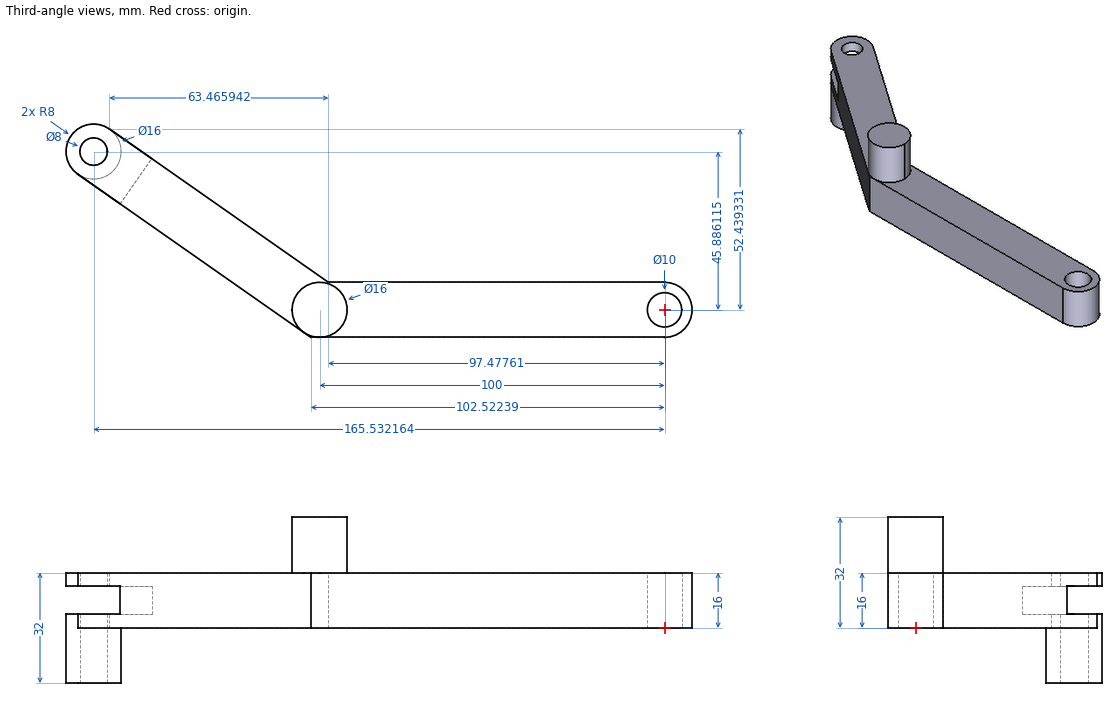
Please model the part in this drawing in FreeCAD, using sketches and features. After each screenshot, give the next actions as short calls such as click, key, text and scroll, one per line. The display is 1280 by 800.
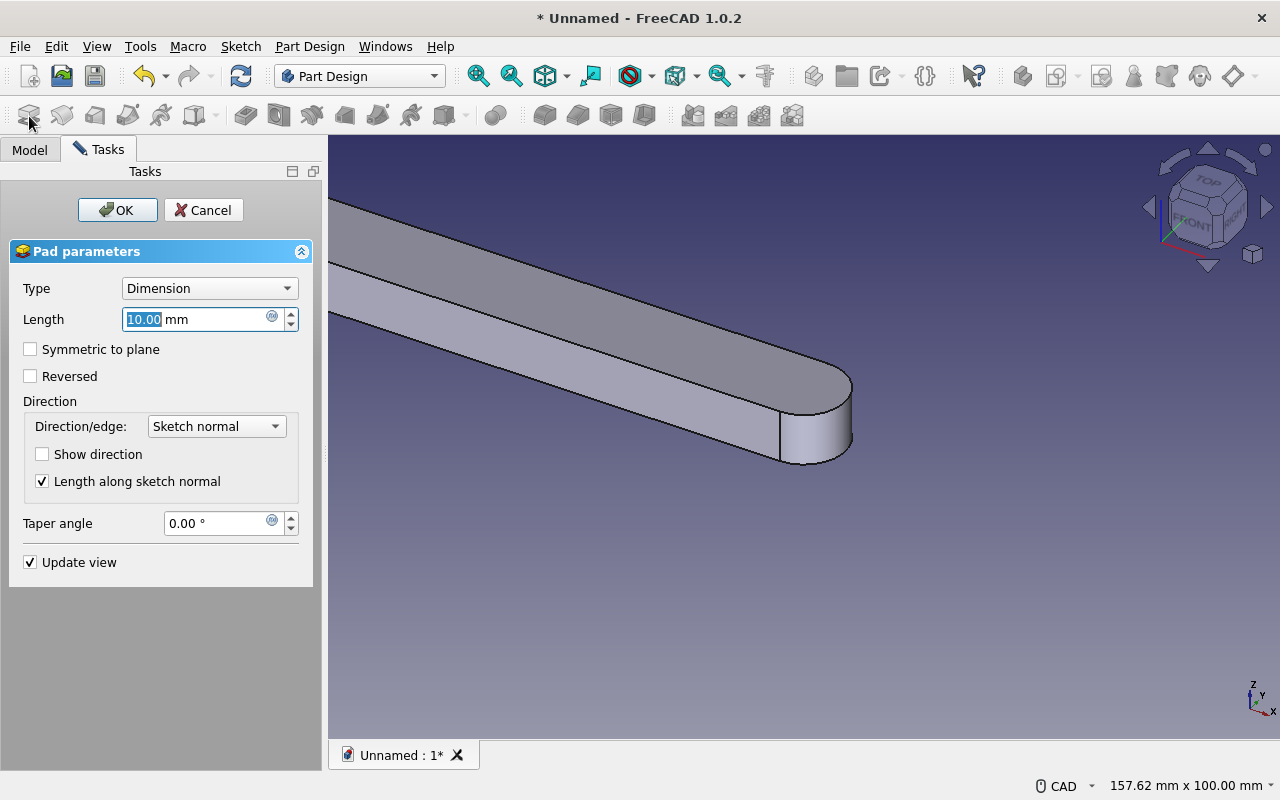
text(16)
key(Tab)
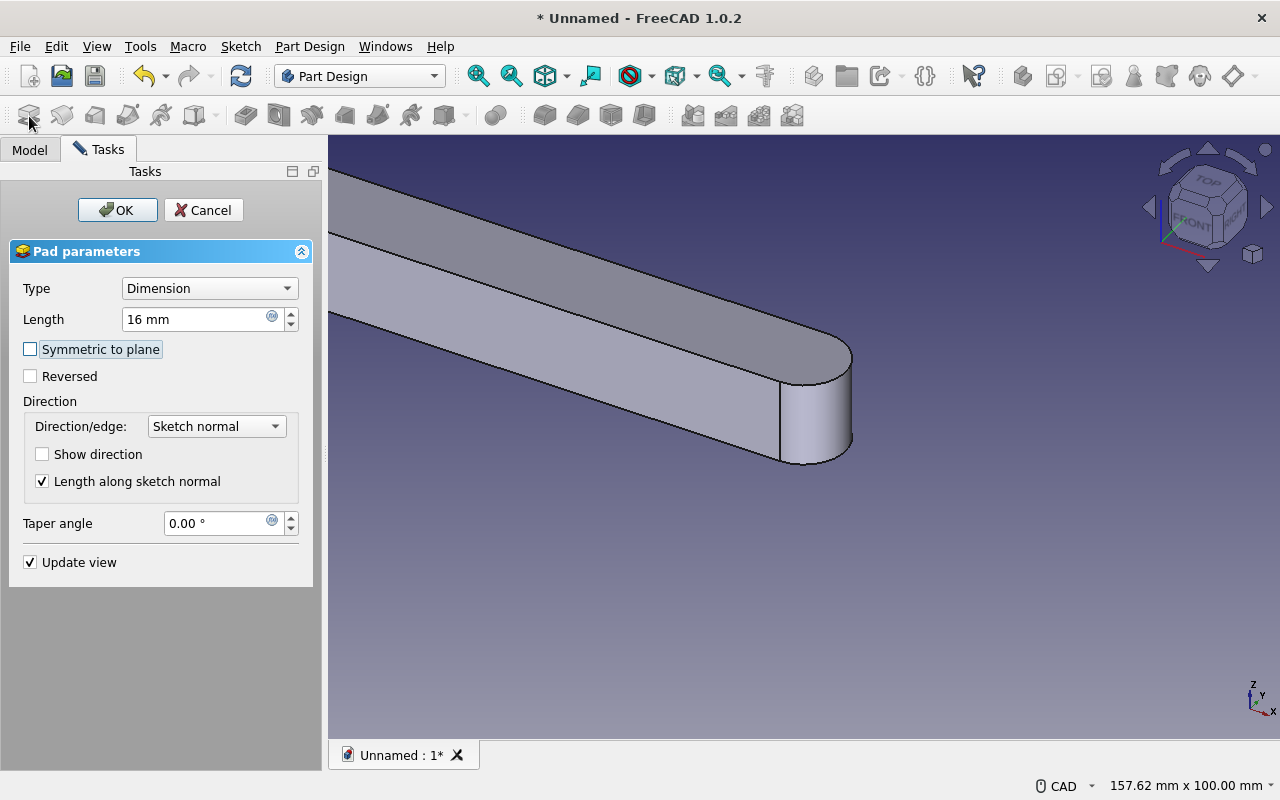
click(118, 210)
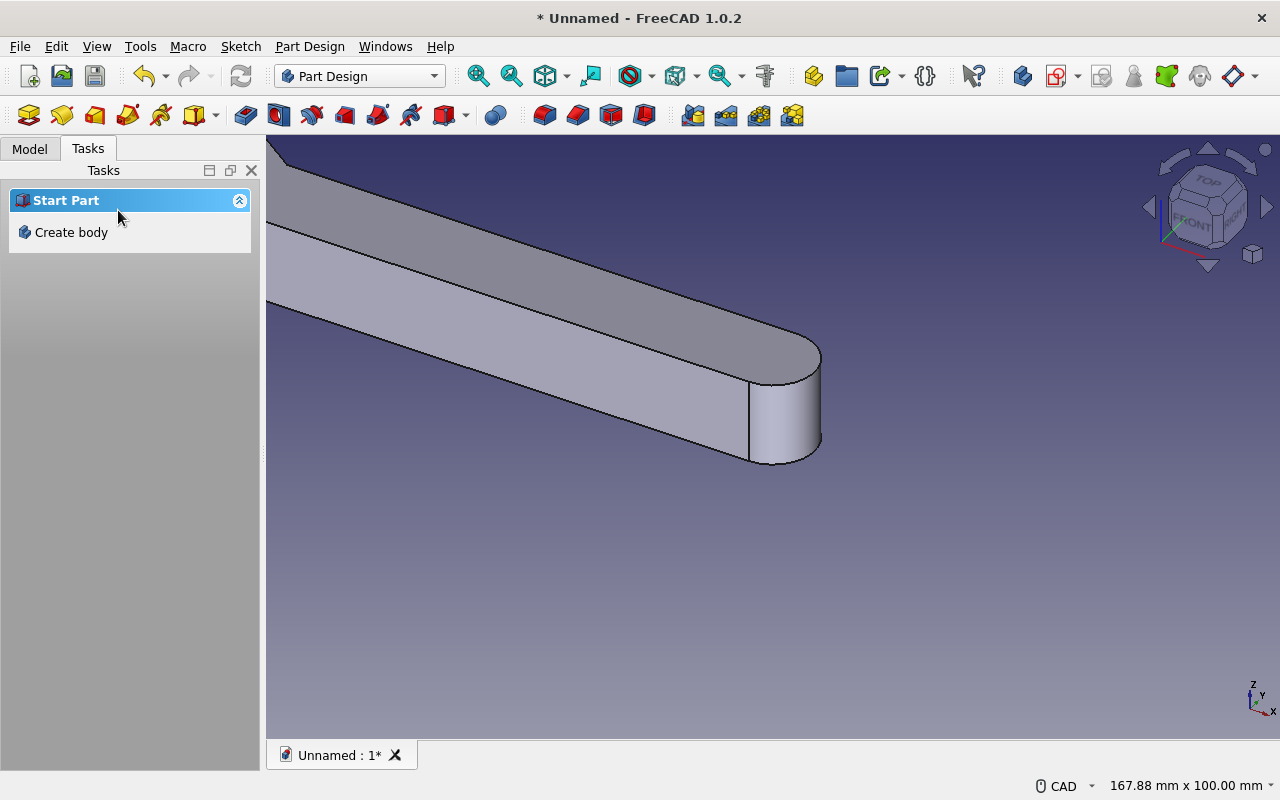
click(479, 76)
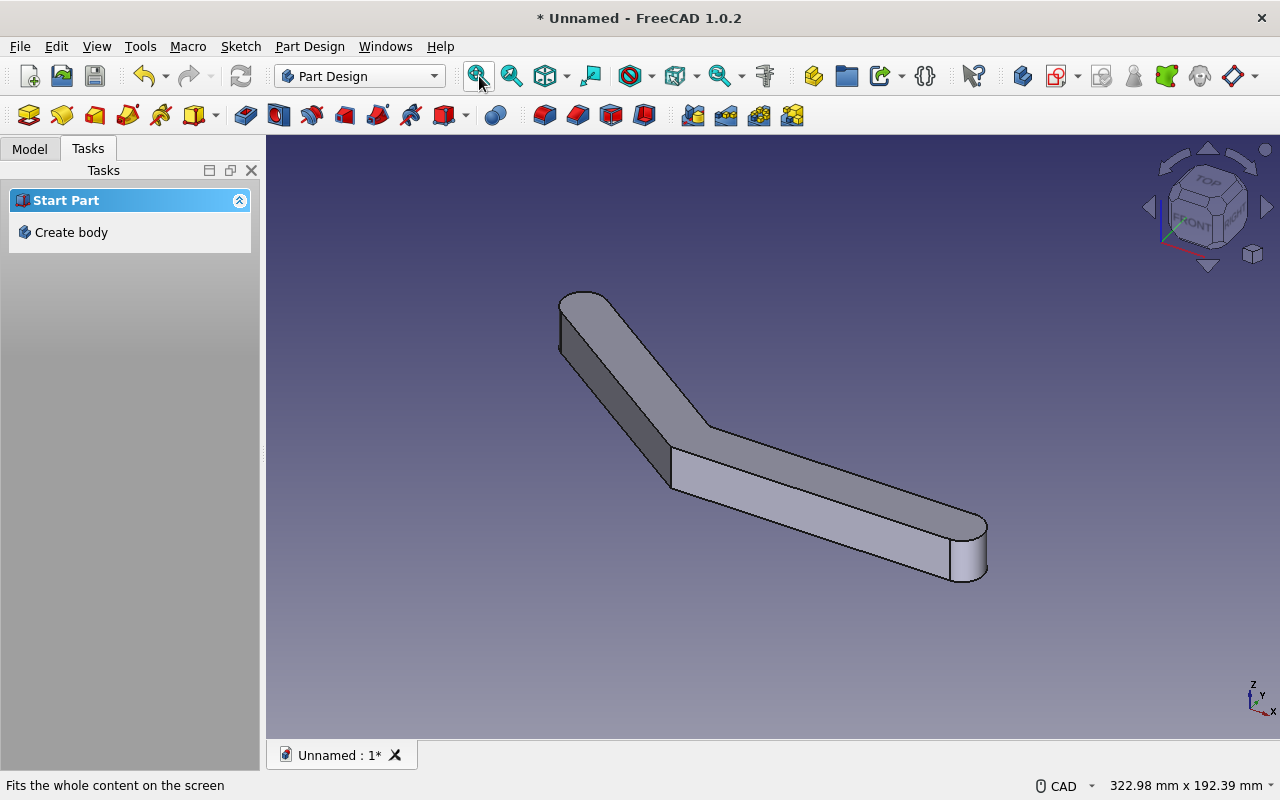
click(675, 420)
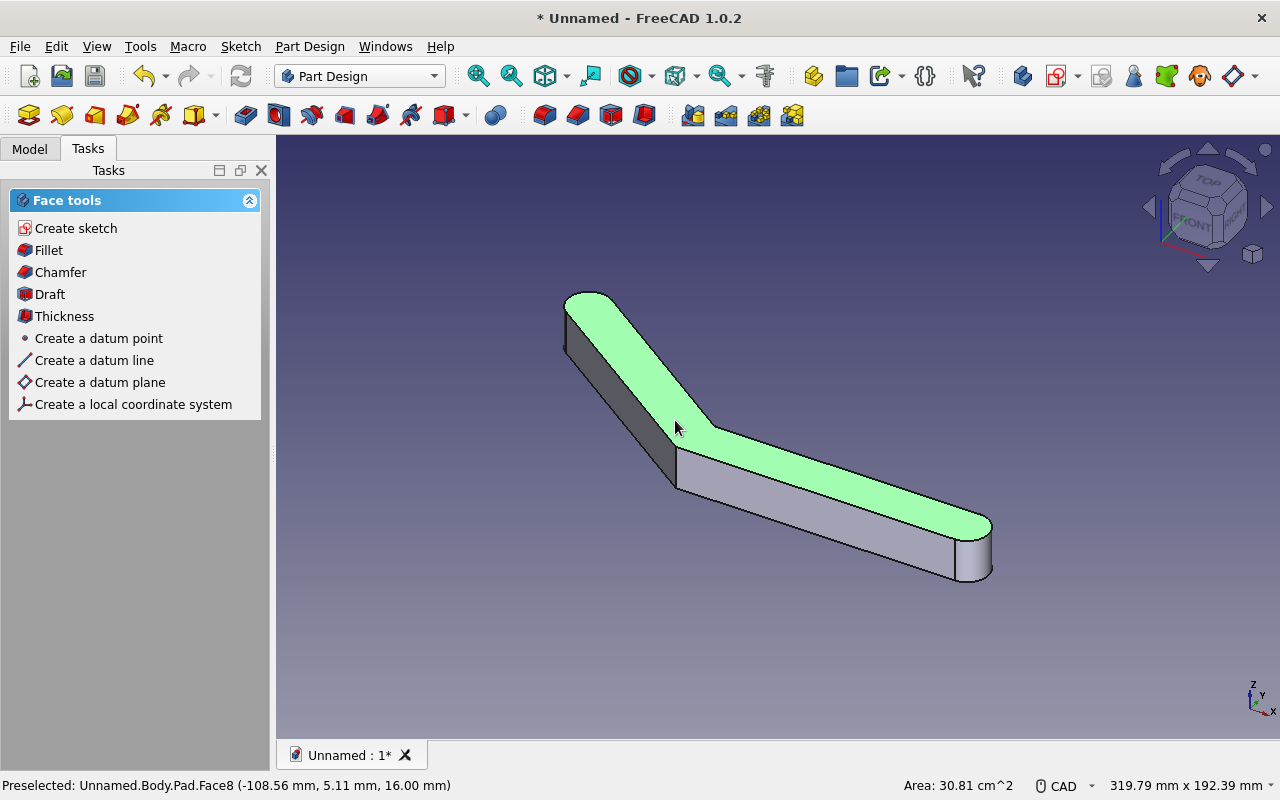
click(1056, 76)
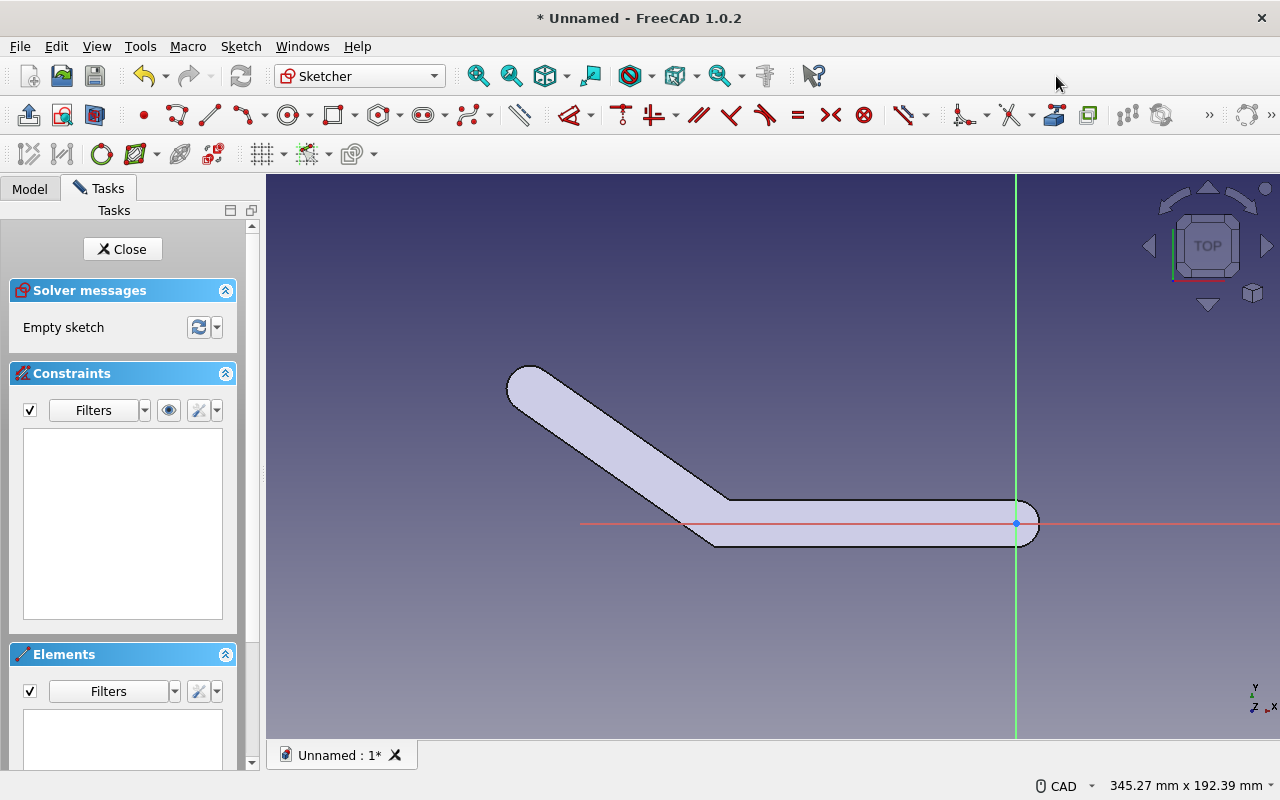
scroll(1041, 529, up, 13)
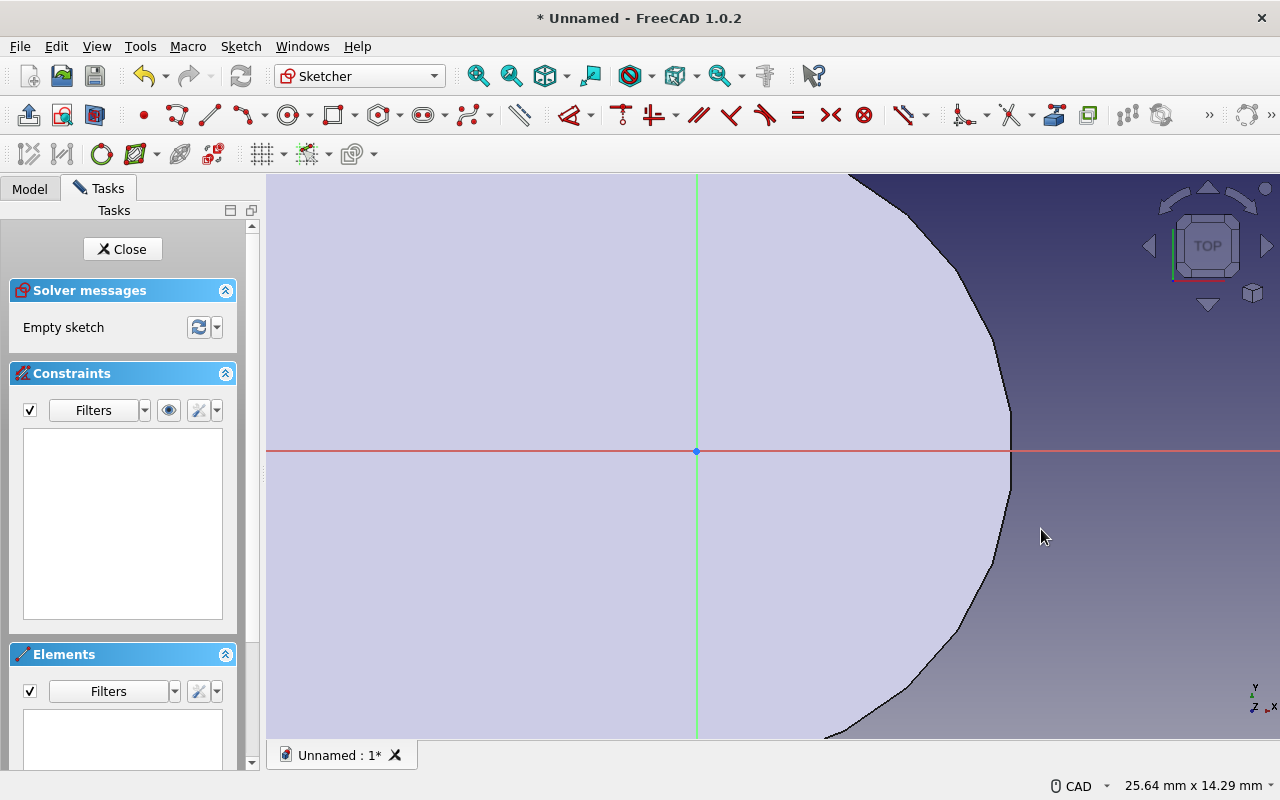
click(288, 116)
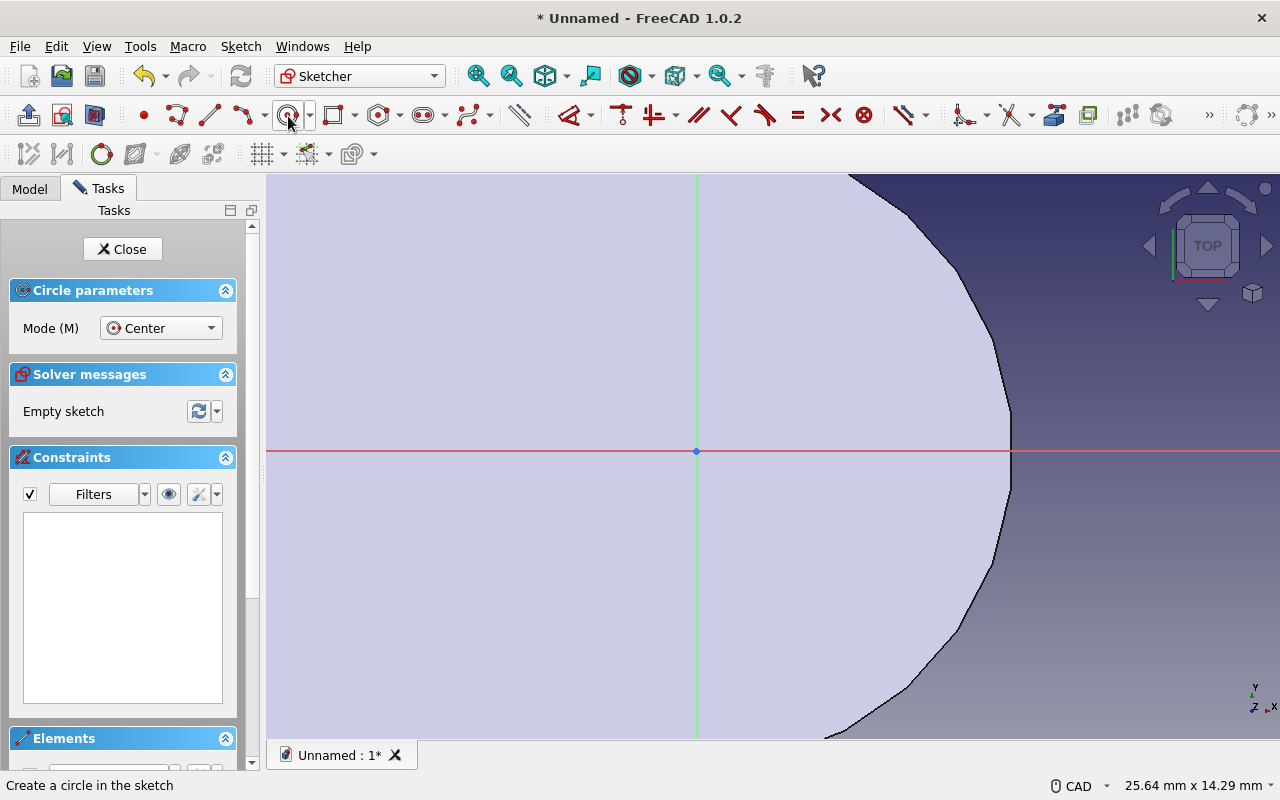
click(697, 451)
click(837, 311)
key(Escape)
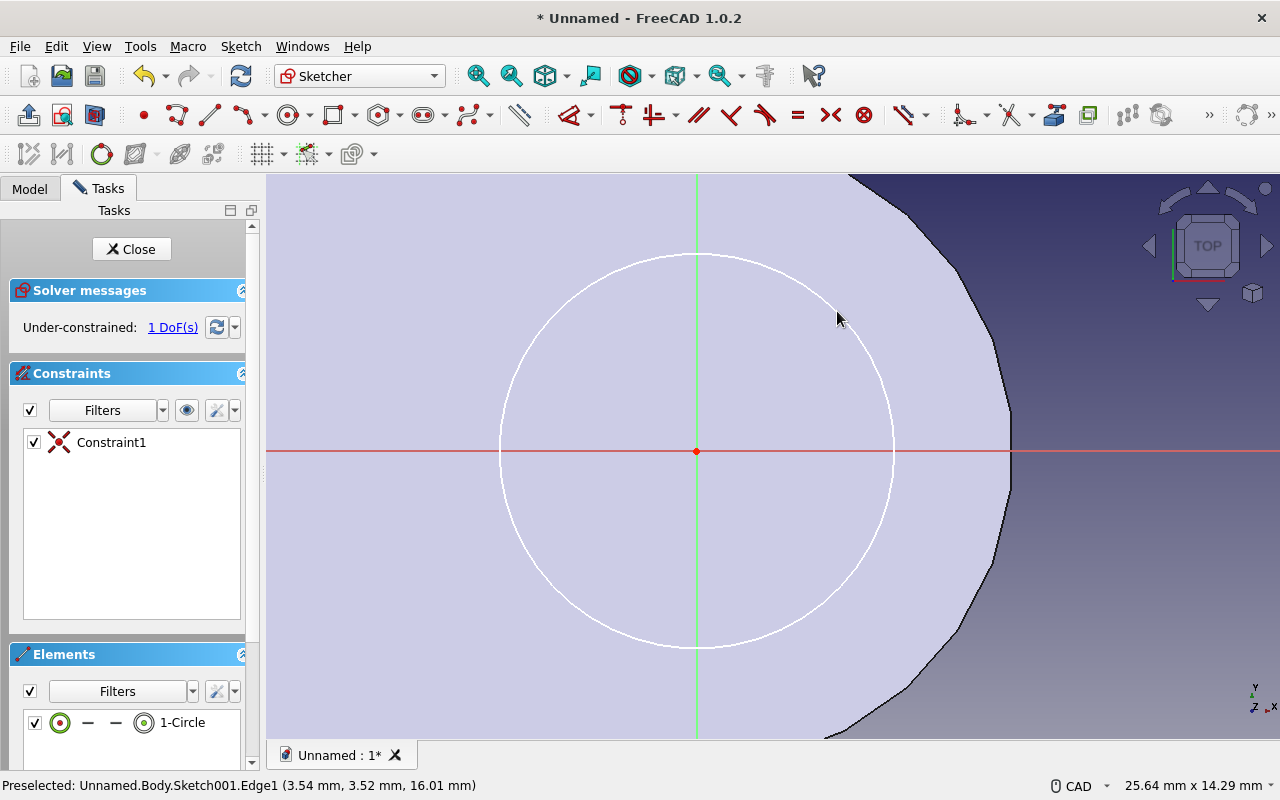
key(d)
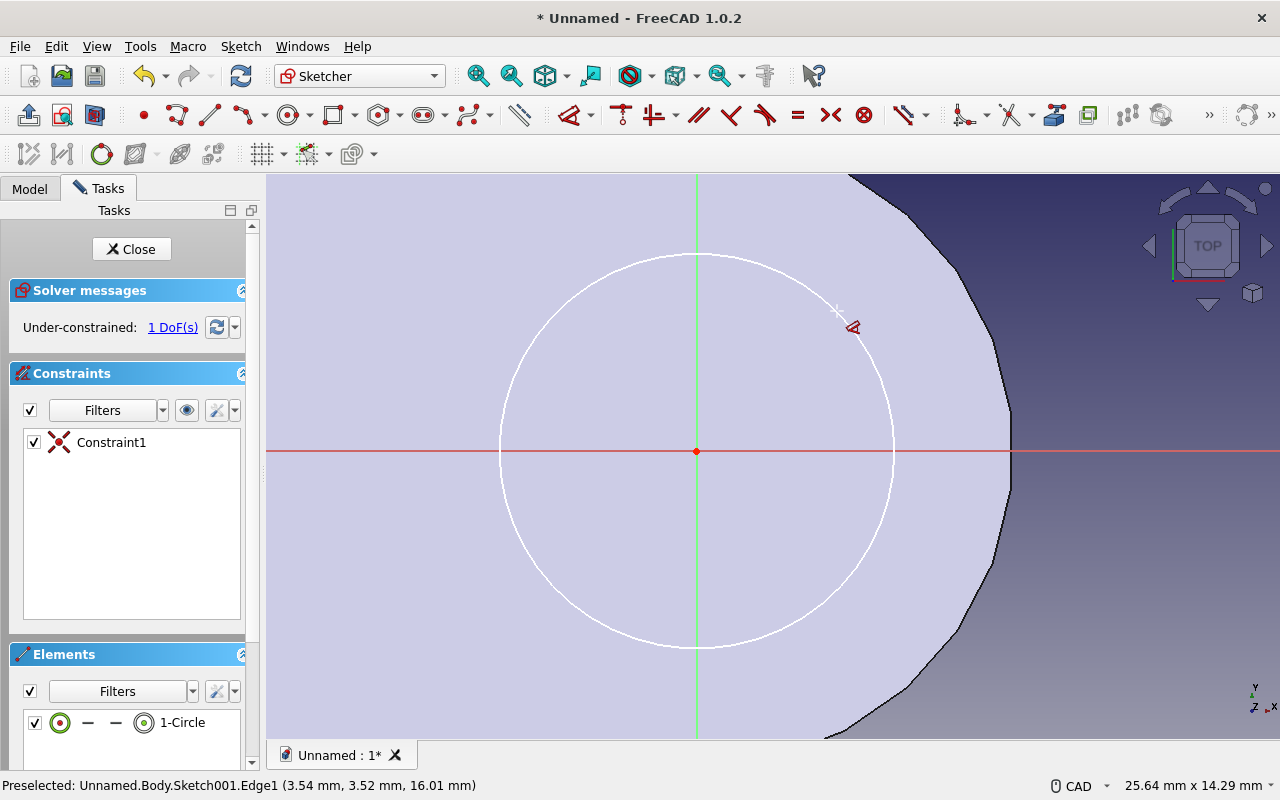
click(836, 311)
click(859, 288)